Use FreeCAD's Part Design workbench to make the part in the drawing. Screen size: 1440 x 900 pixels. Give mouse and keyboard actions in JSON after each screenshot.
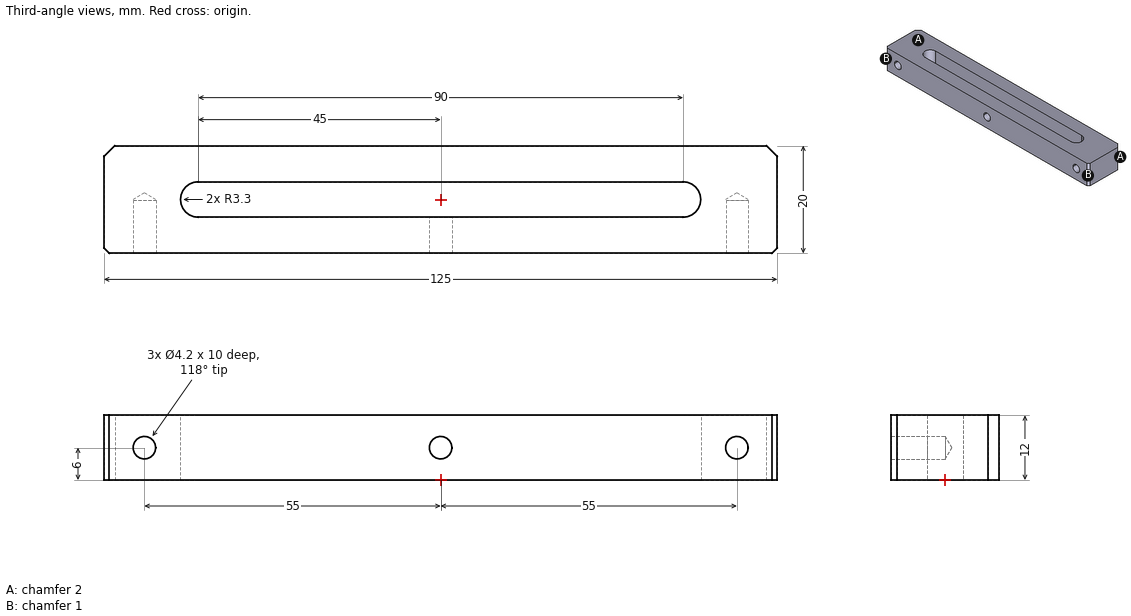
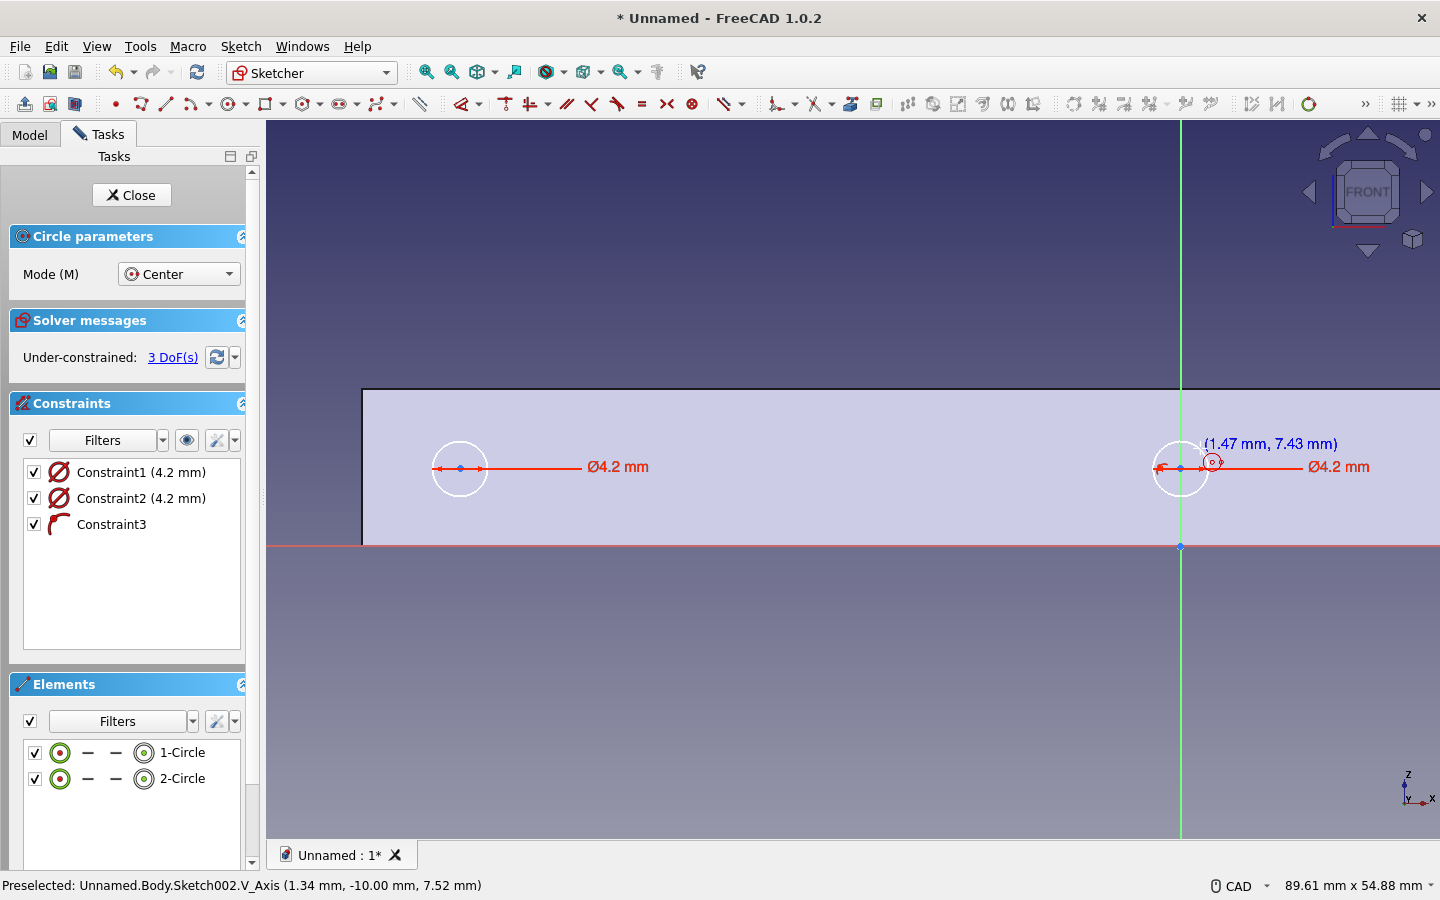
{"action": "scroll", "coordinate": [461, 468], "scroll_direction": "down", "scroll_amount": 4}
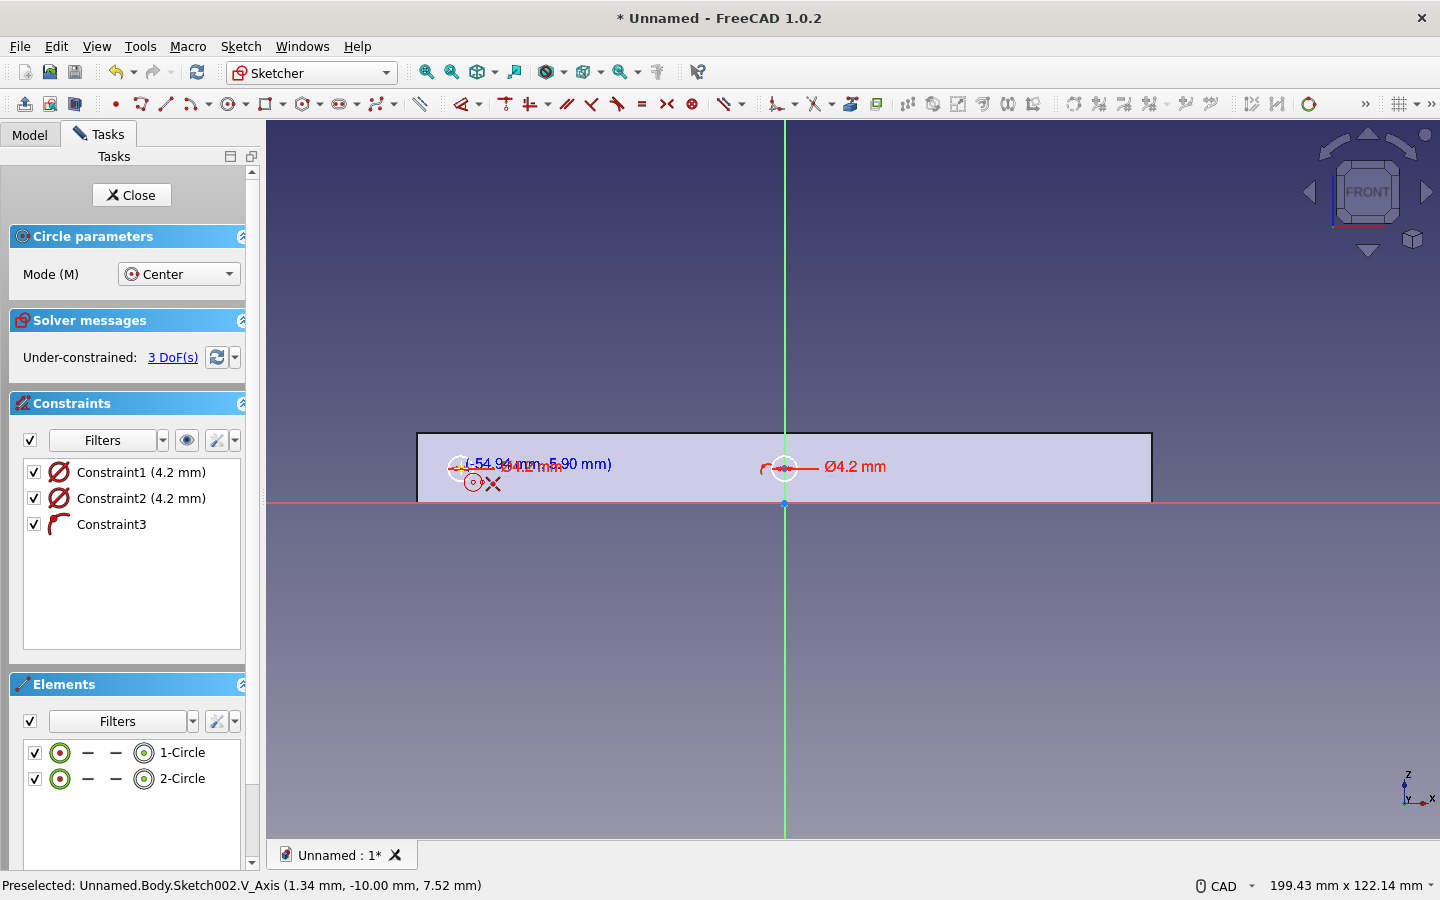
{"action": "scroll", "coordinate": [1108, 468], "scroll_direction": "up", "scroll_amount": 4}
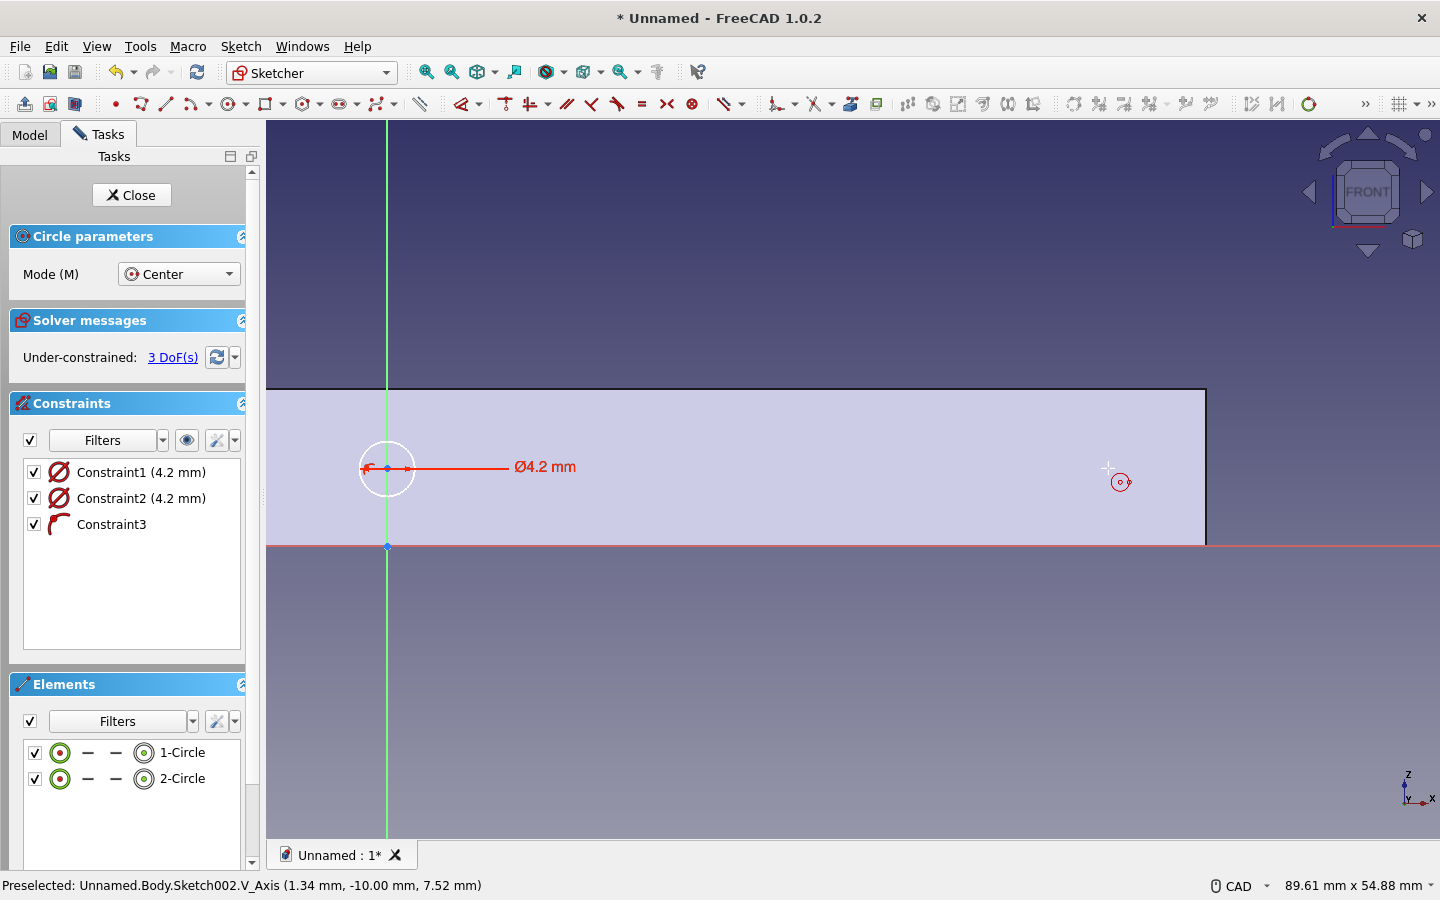
{"action": "left_click", "coordinate": [1108, 468]}
{"action": "mouse_move", "coordinate": [1127, 448]}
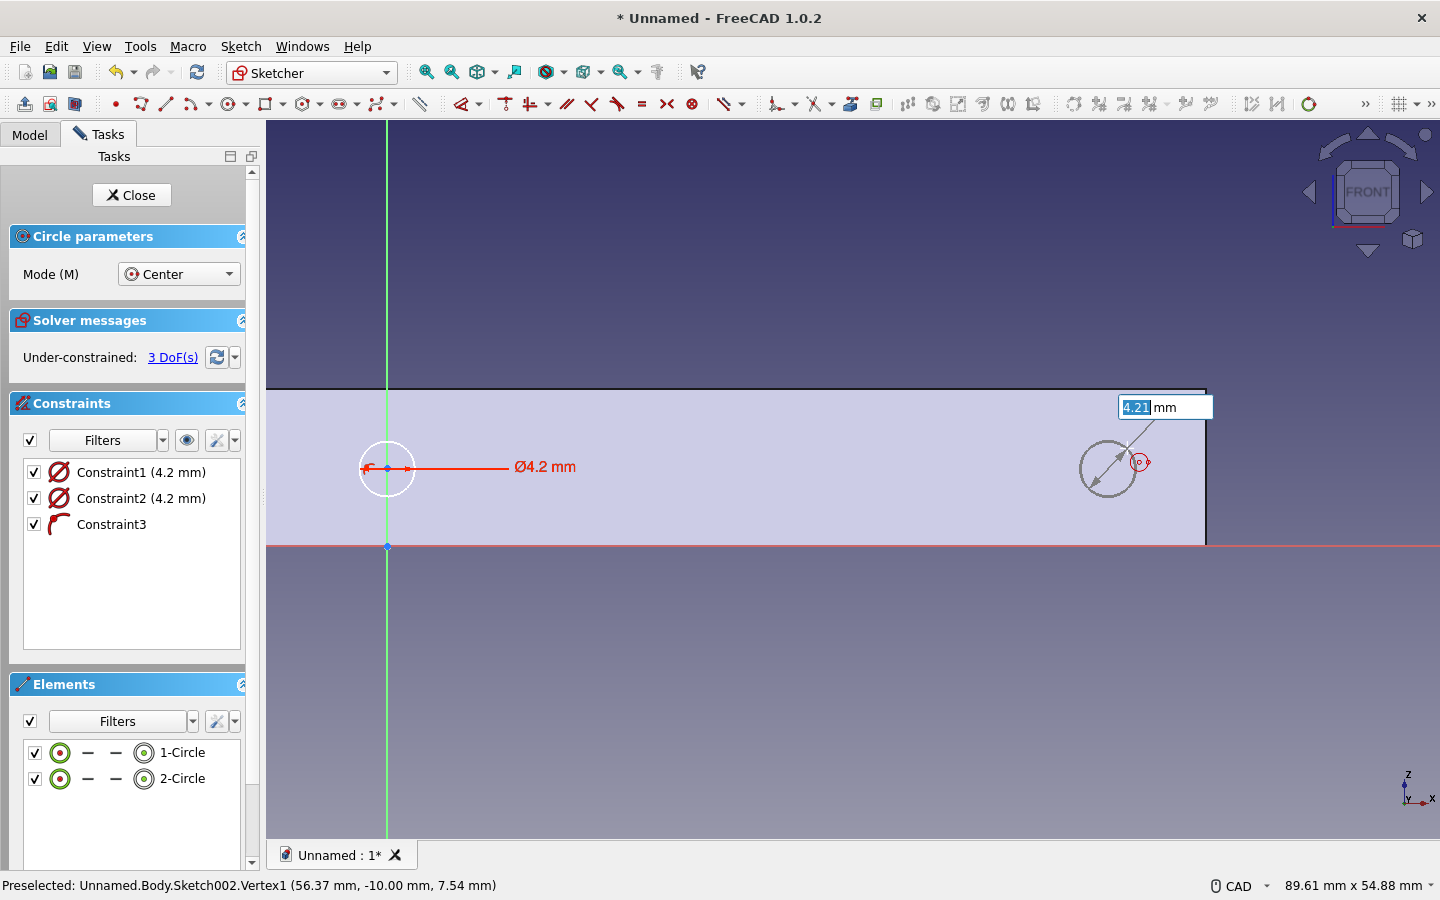
{"action": "type", "text": "4.2"}
{"action": "key", "text": "Return"}
{"action": "key", "text": "Escape"}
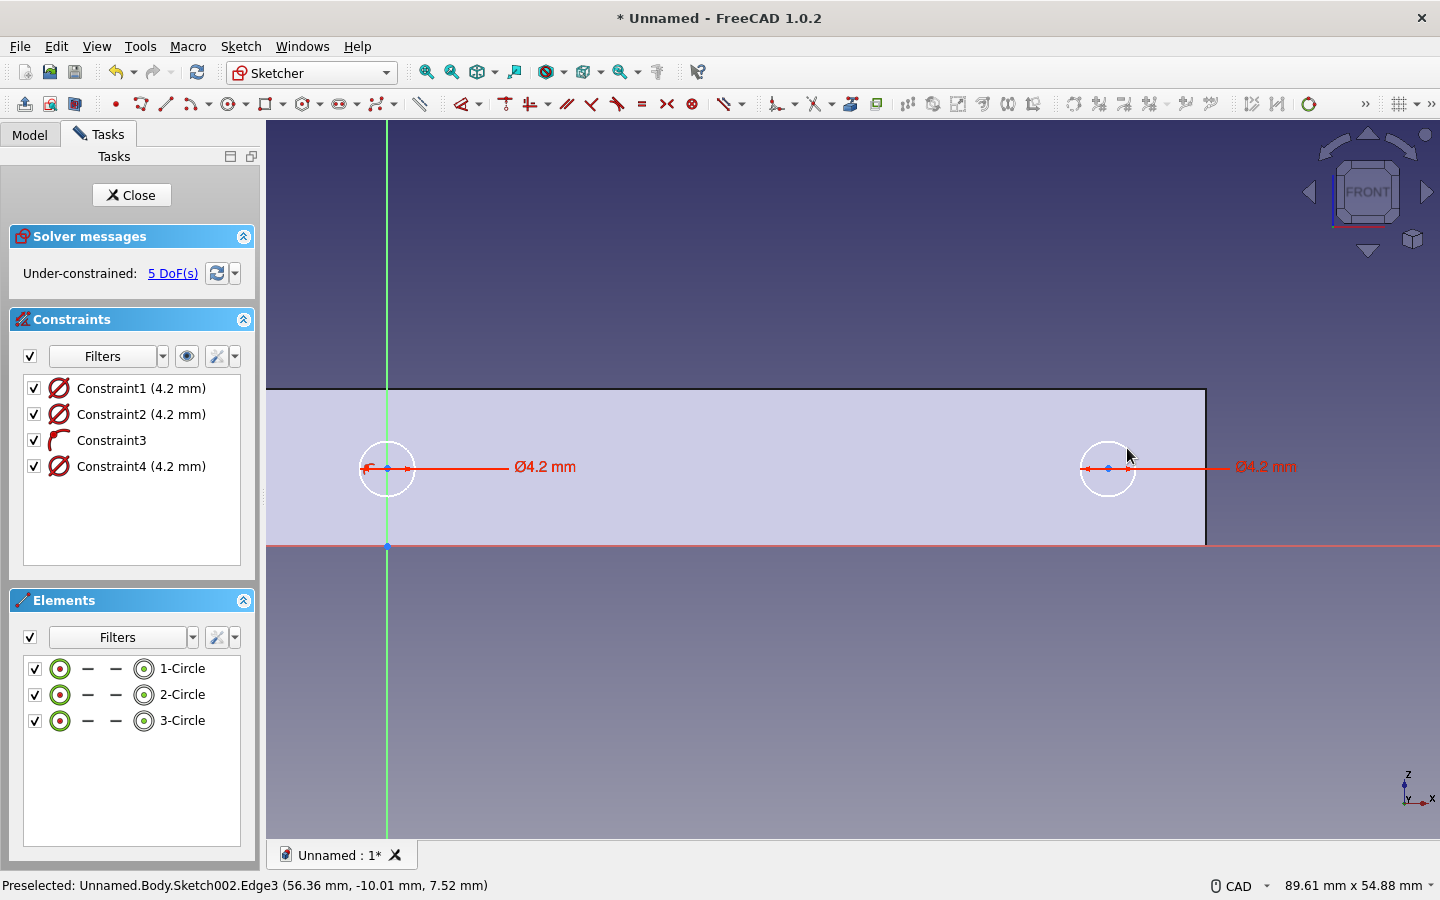
{"action": "scroll", "coordinate": [1109, 468], "scroll_direction": "down", "scroll_amount": 4}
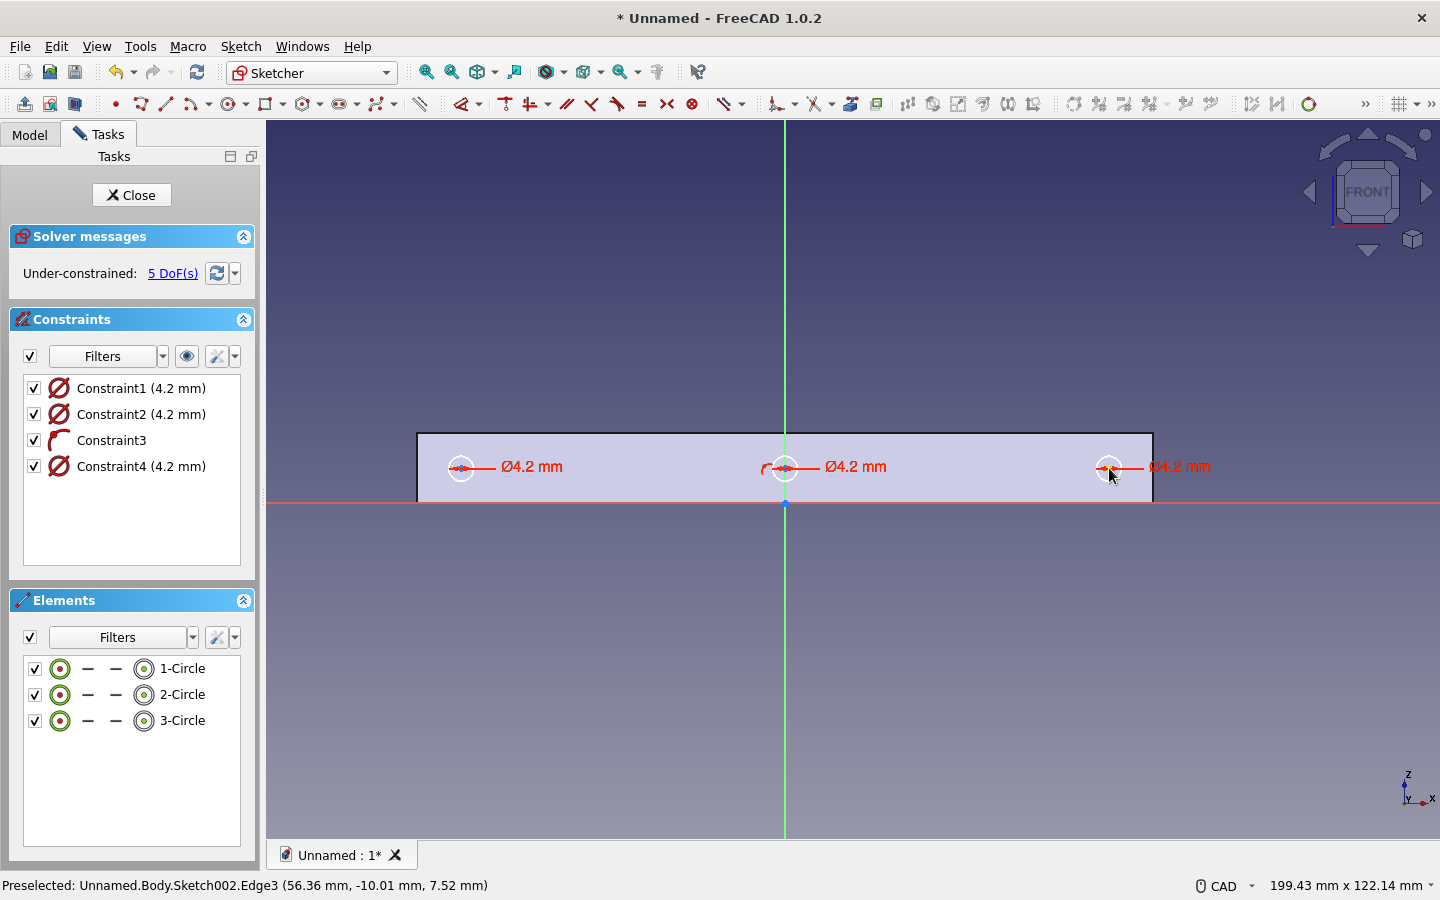
{"action": "left_click", "coordinate": [461, 469]}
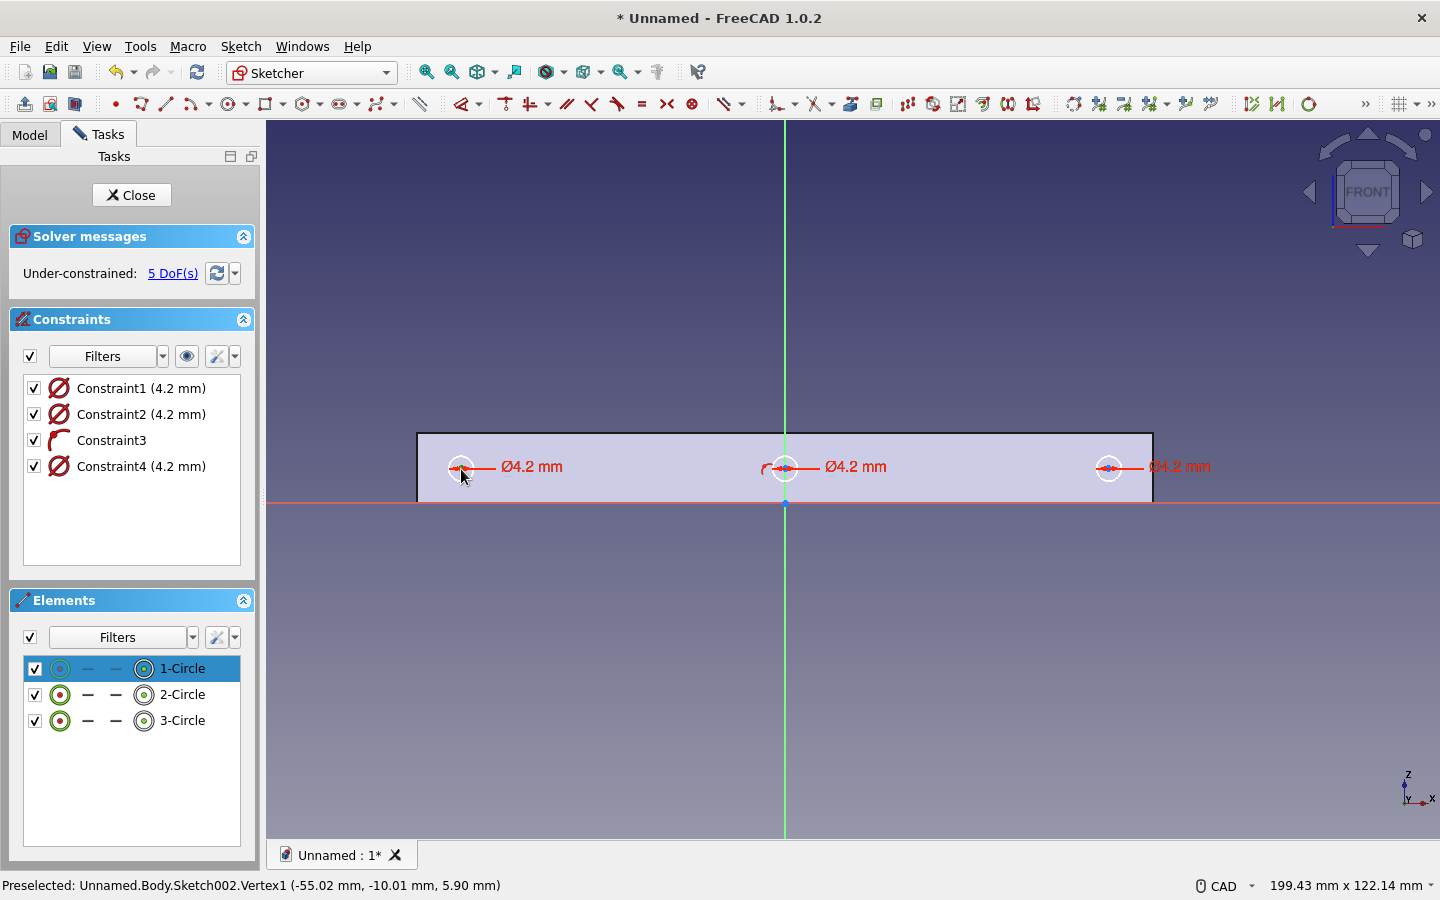
{"action": "left_click", "coordinate": [785, 469]}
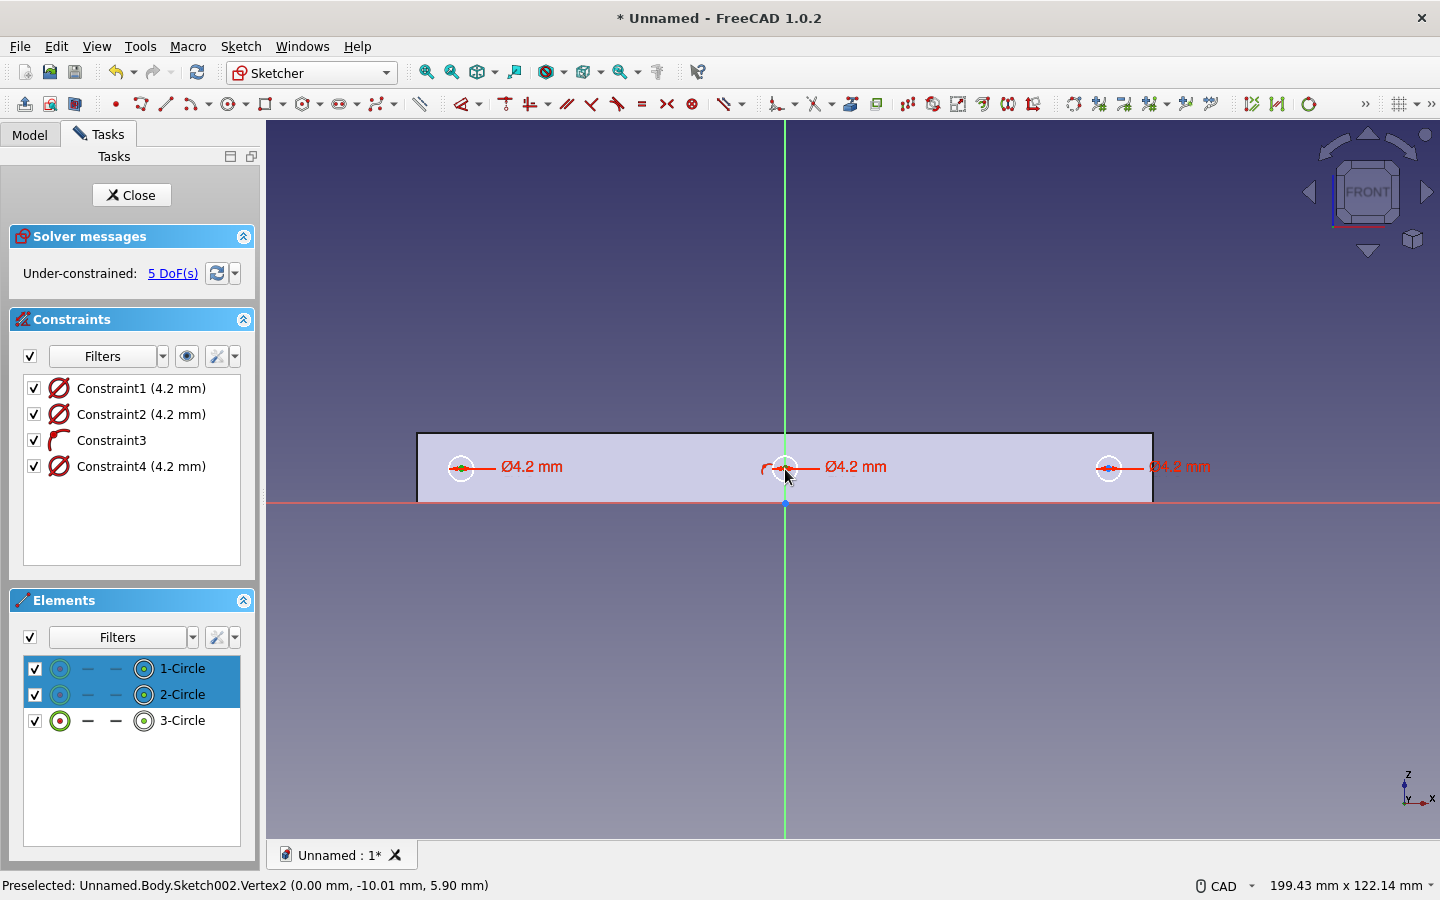
{"action": "key", "text": "h"}